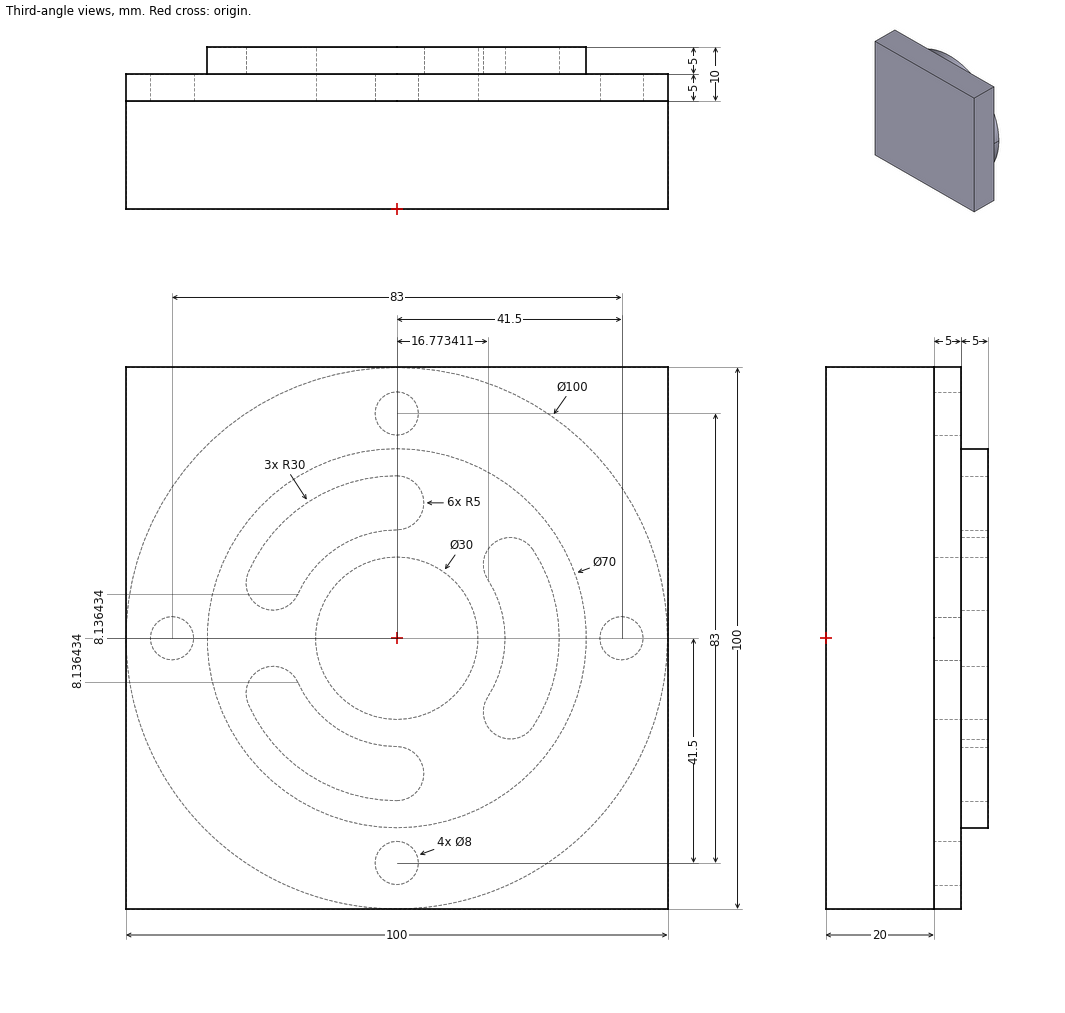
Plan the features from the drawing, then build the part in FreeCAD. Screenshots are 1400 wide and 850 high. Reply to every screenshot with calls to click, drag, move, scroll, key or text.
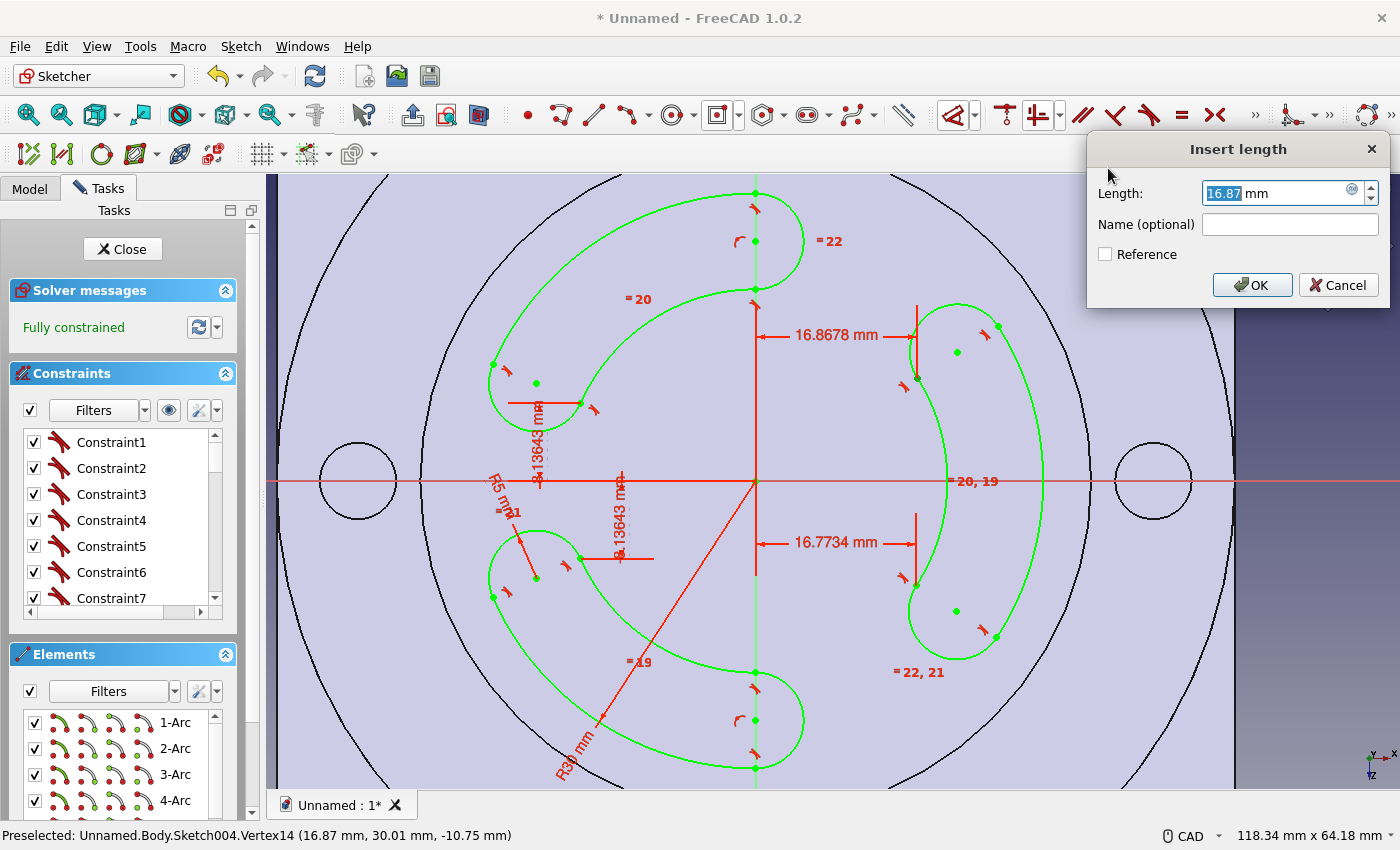
text(16.773411)
key(Return)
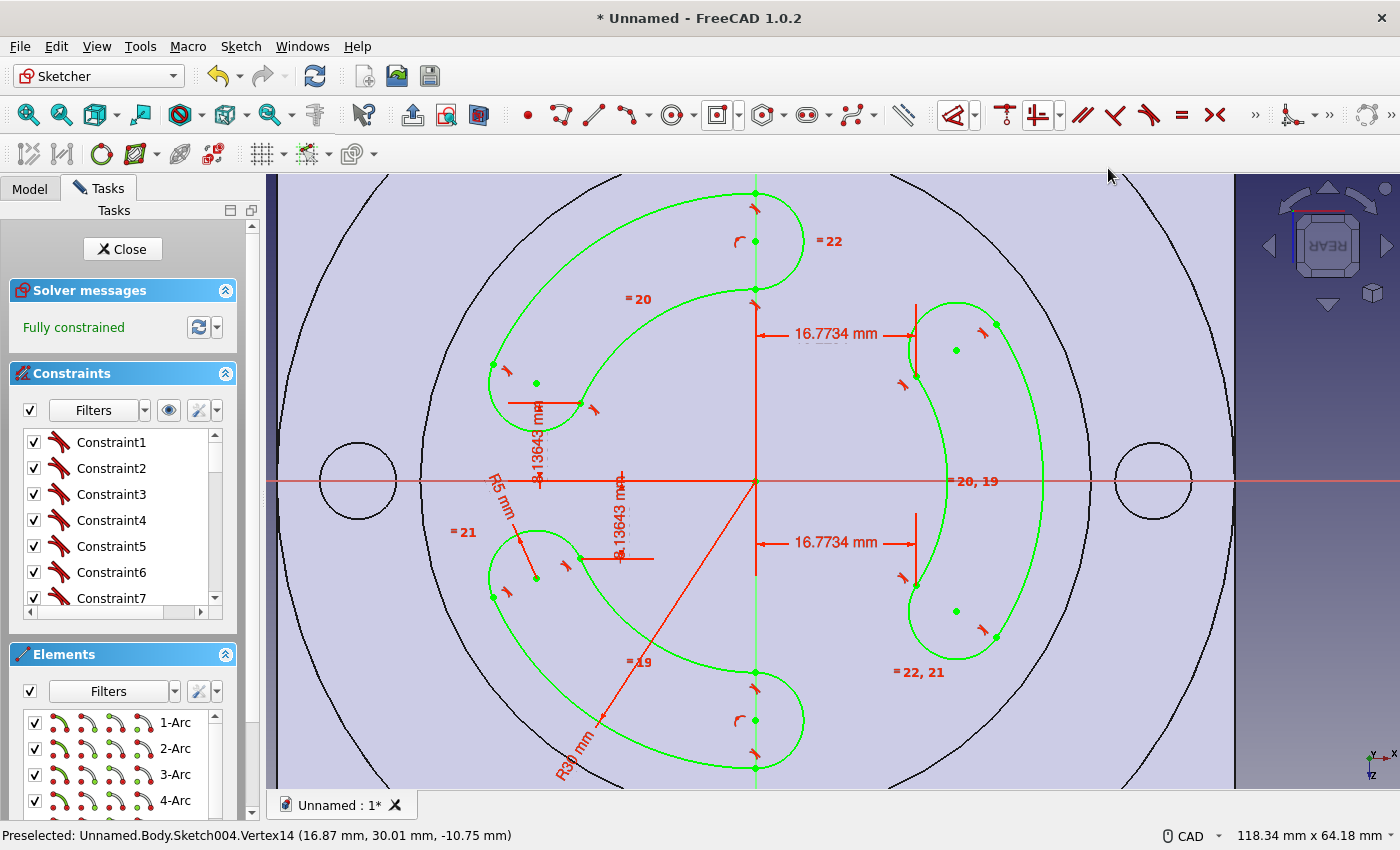
click(123, 249)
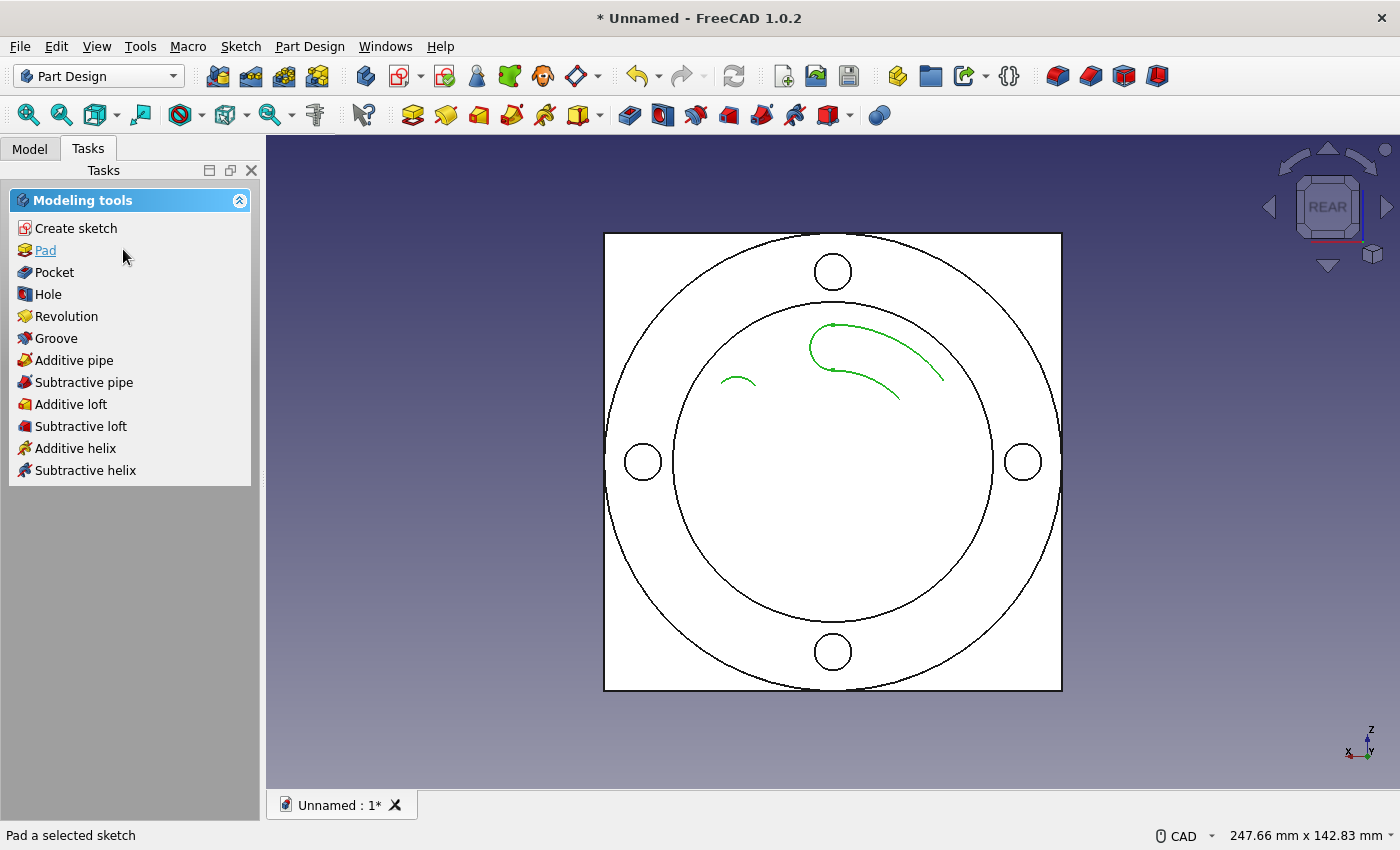
click(630, 116)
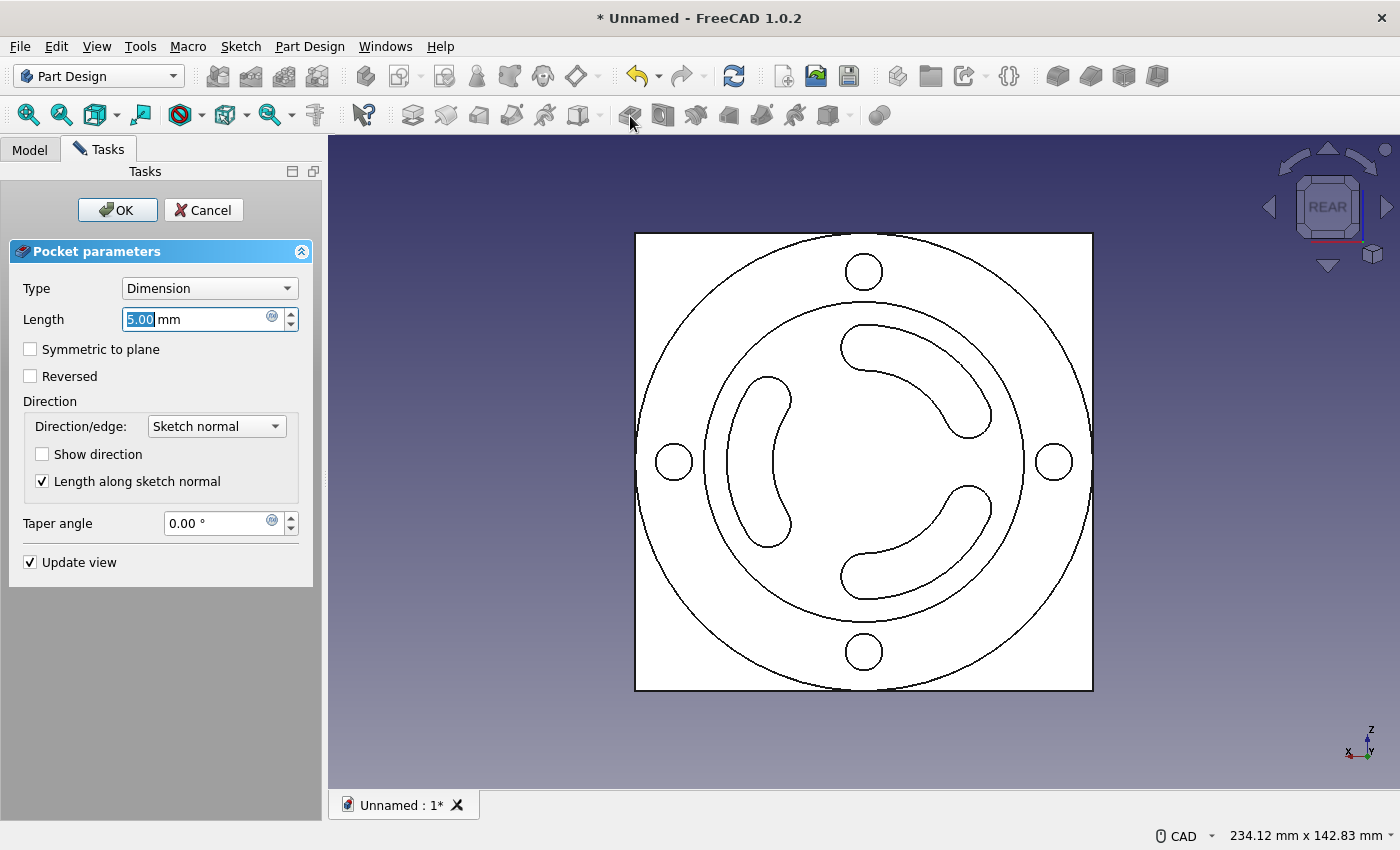
text(5)
key(Tab)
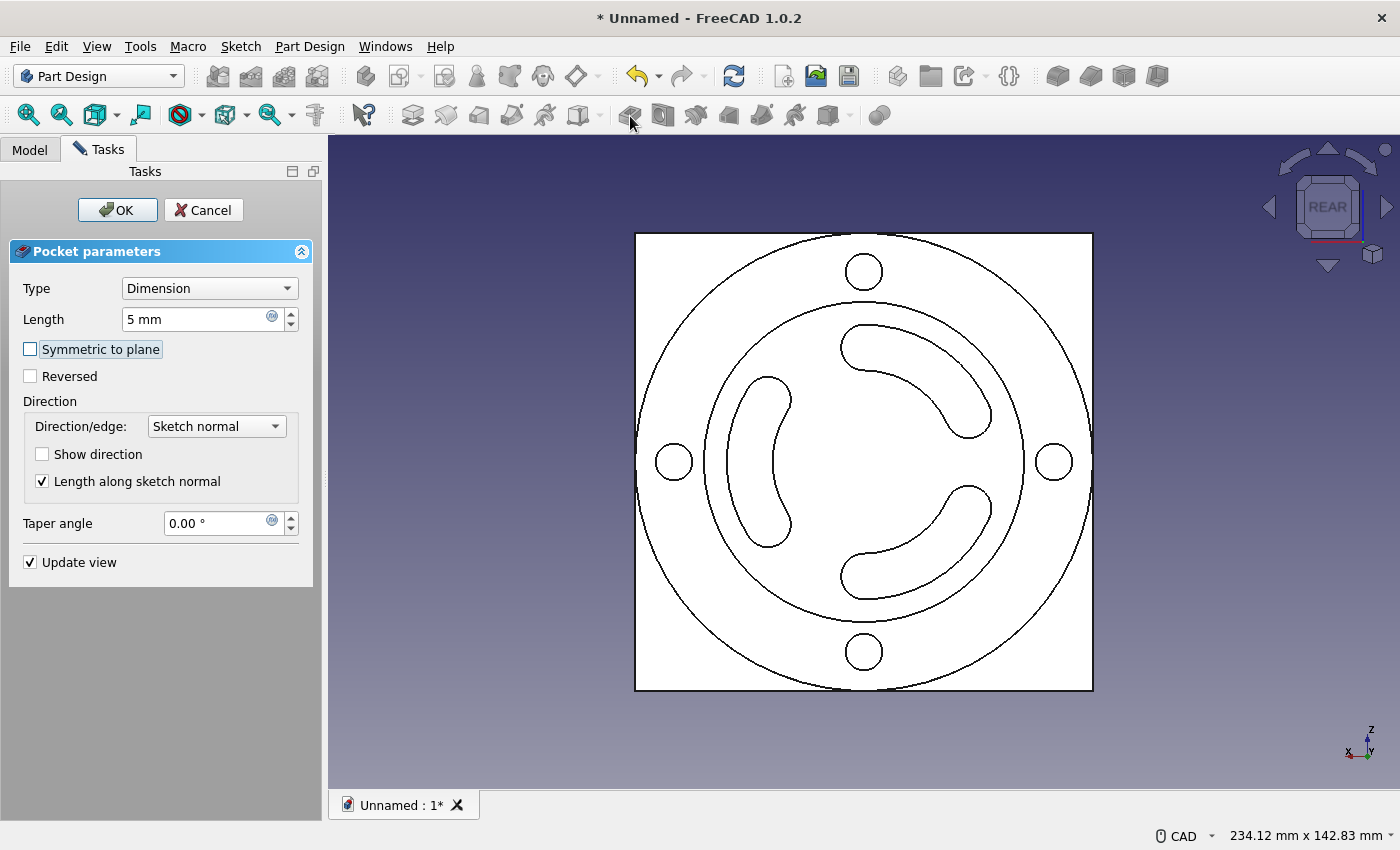
click(118, 210)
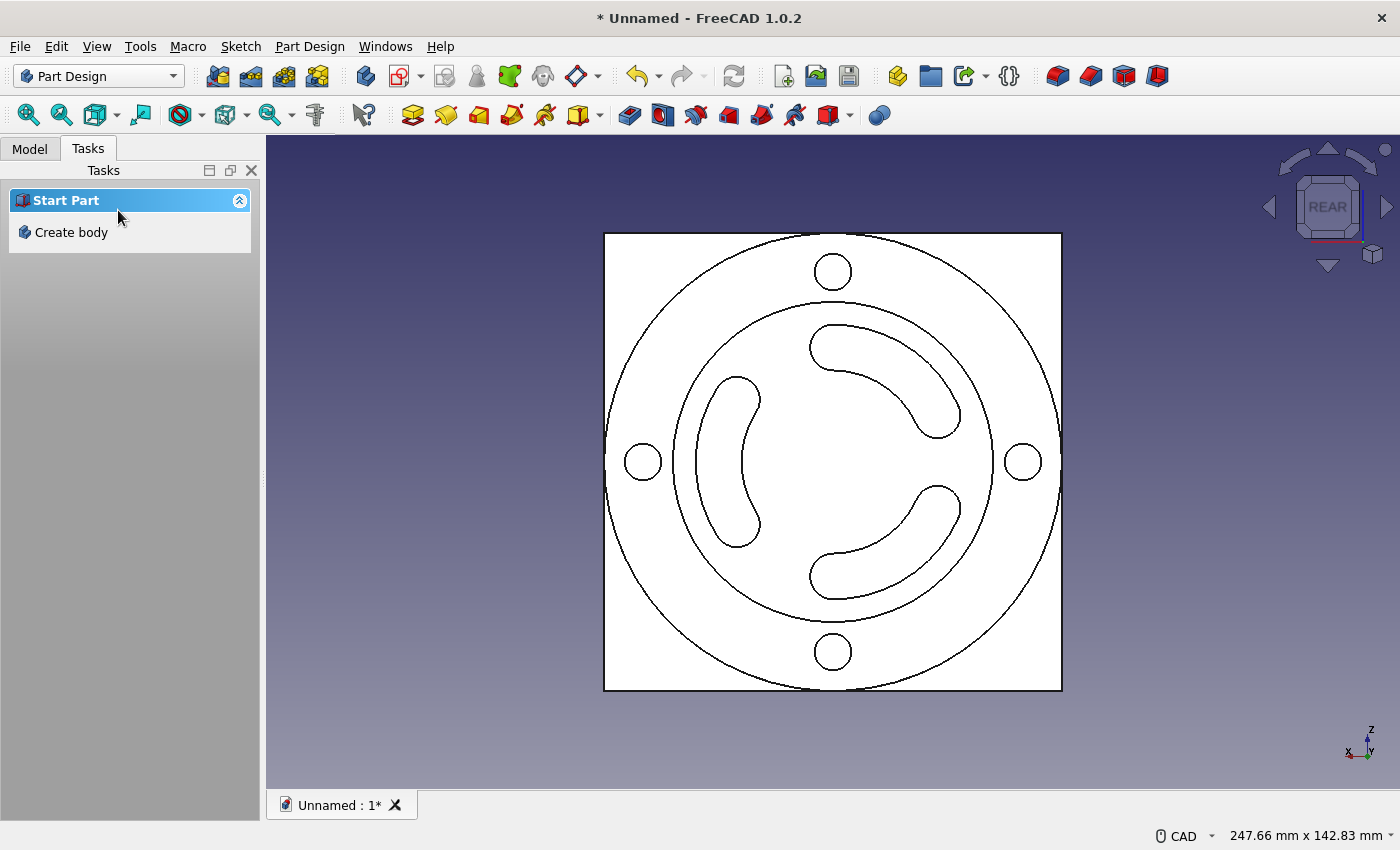
click(833, 461)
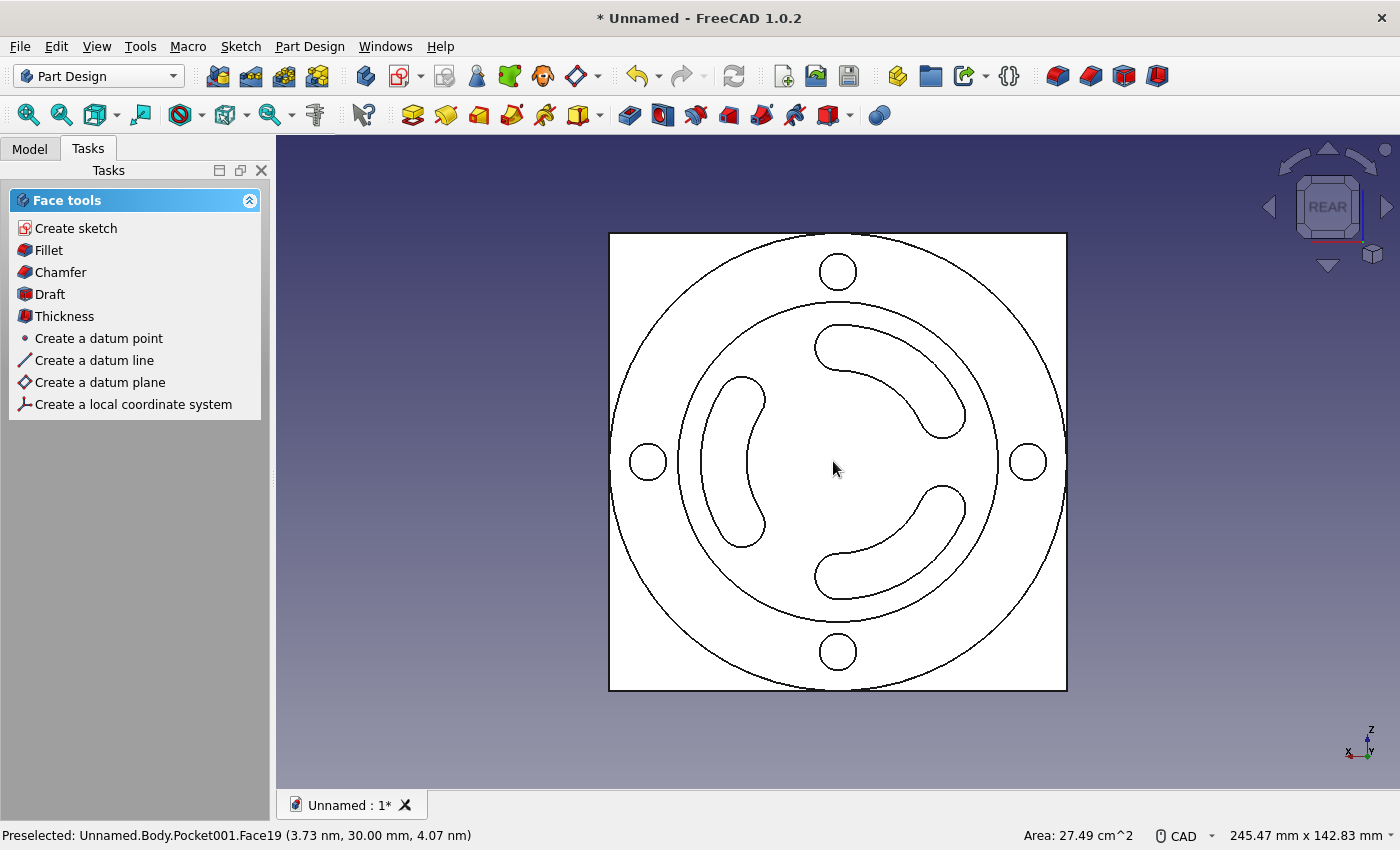
click(398, 76)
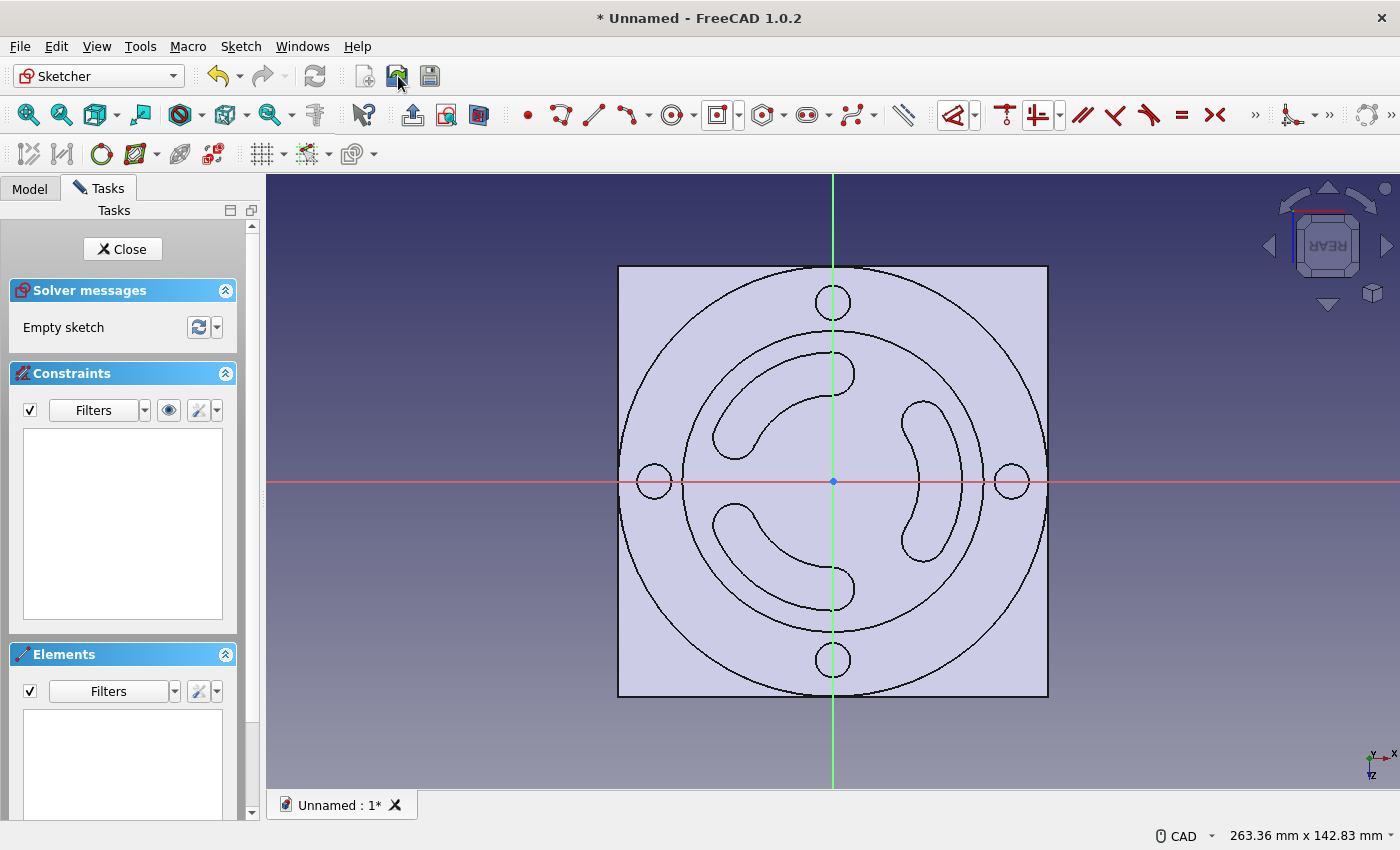
scroll(863, 481, up, 6)